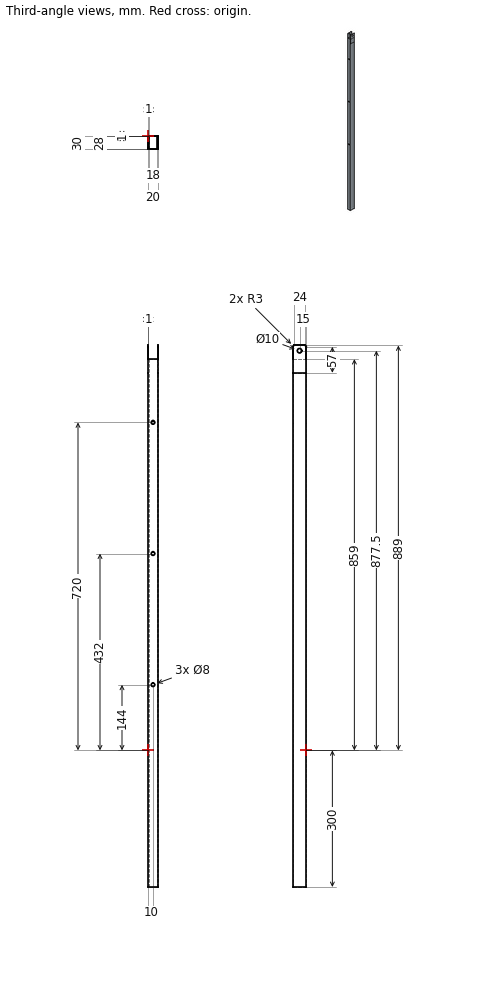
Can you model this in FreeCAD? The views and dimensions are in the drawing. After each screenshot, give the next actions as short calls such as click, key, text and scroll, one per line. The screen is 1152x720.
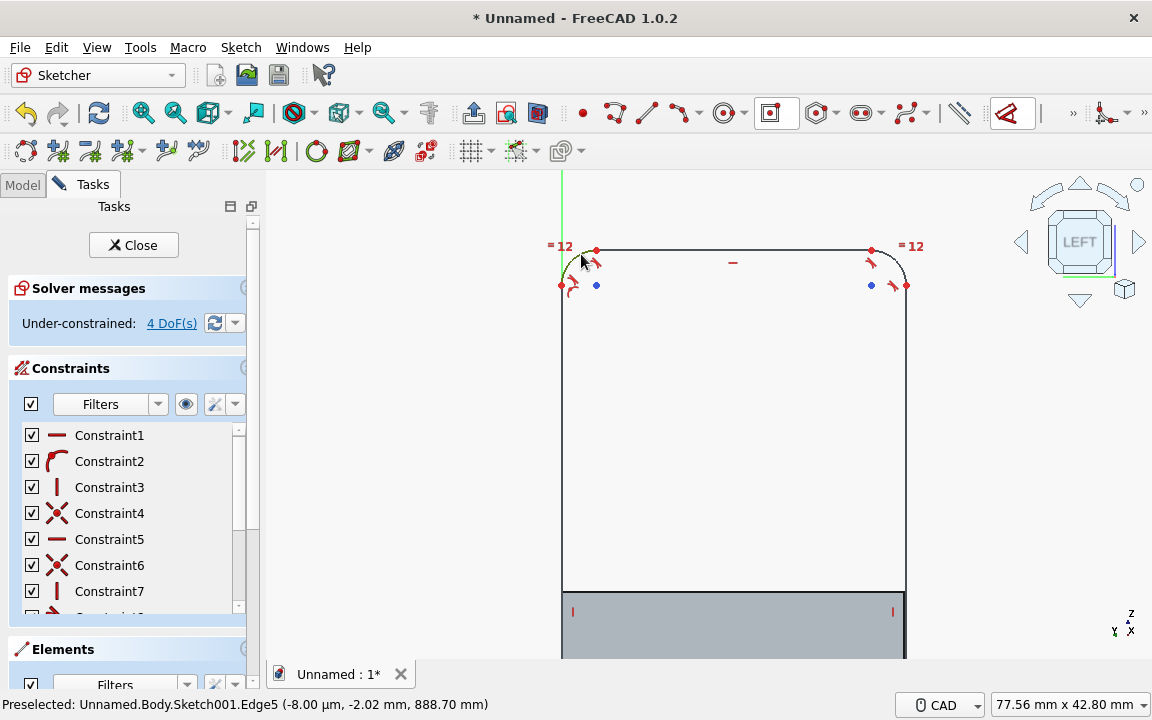
key(k)
key(r)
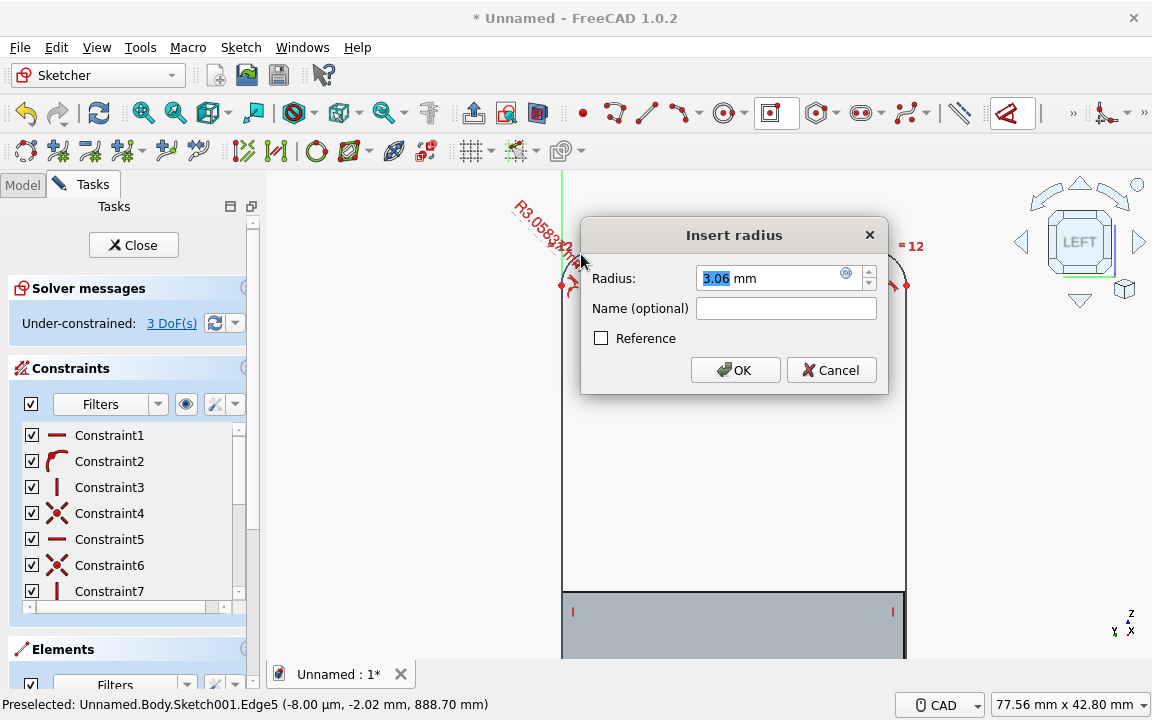
text(3)
key(Return)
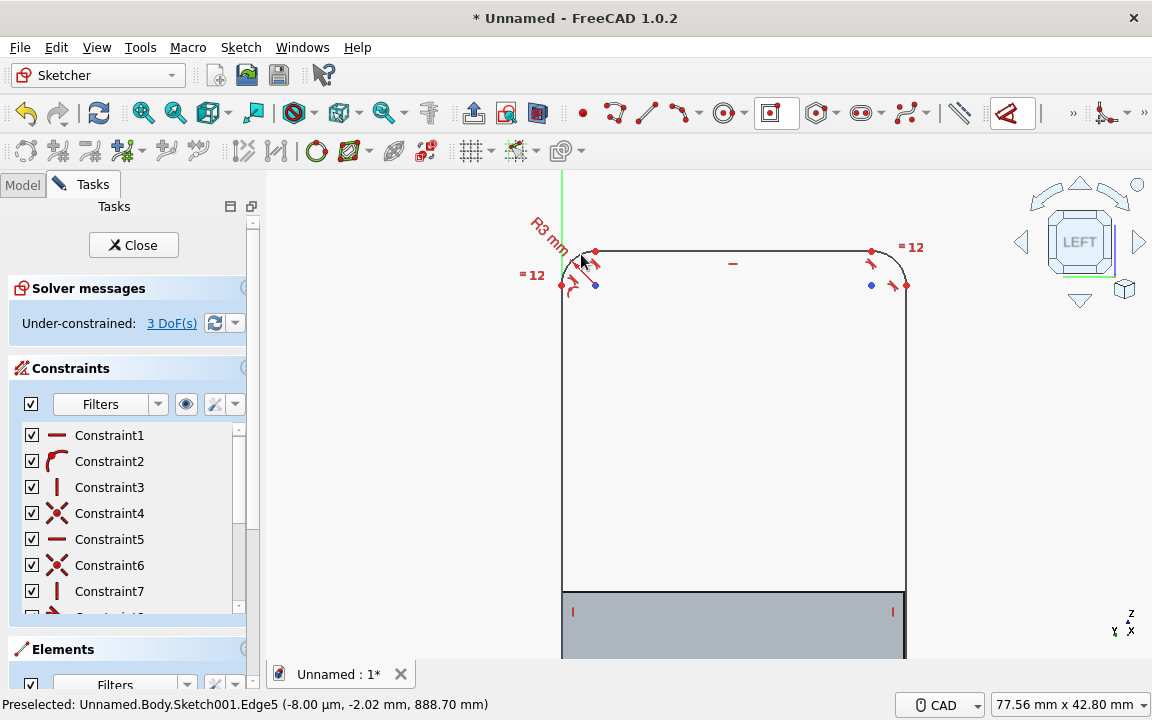
click(789, 251)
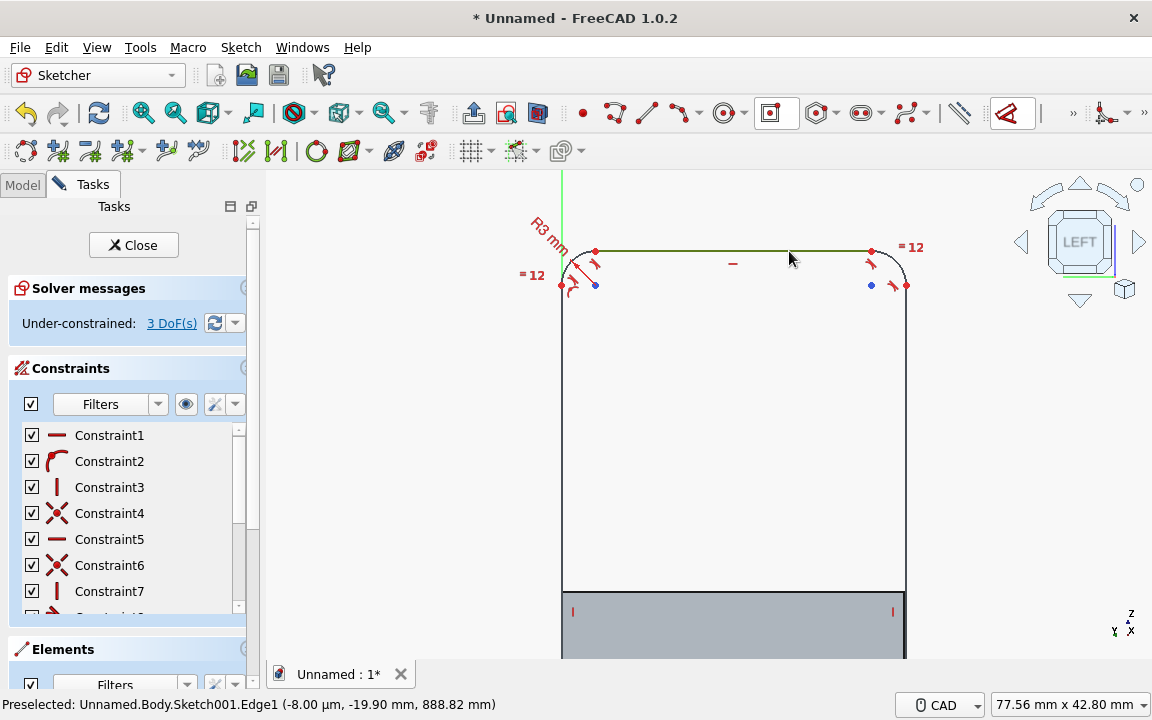
click(1030, 114)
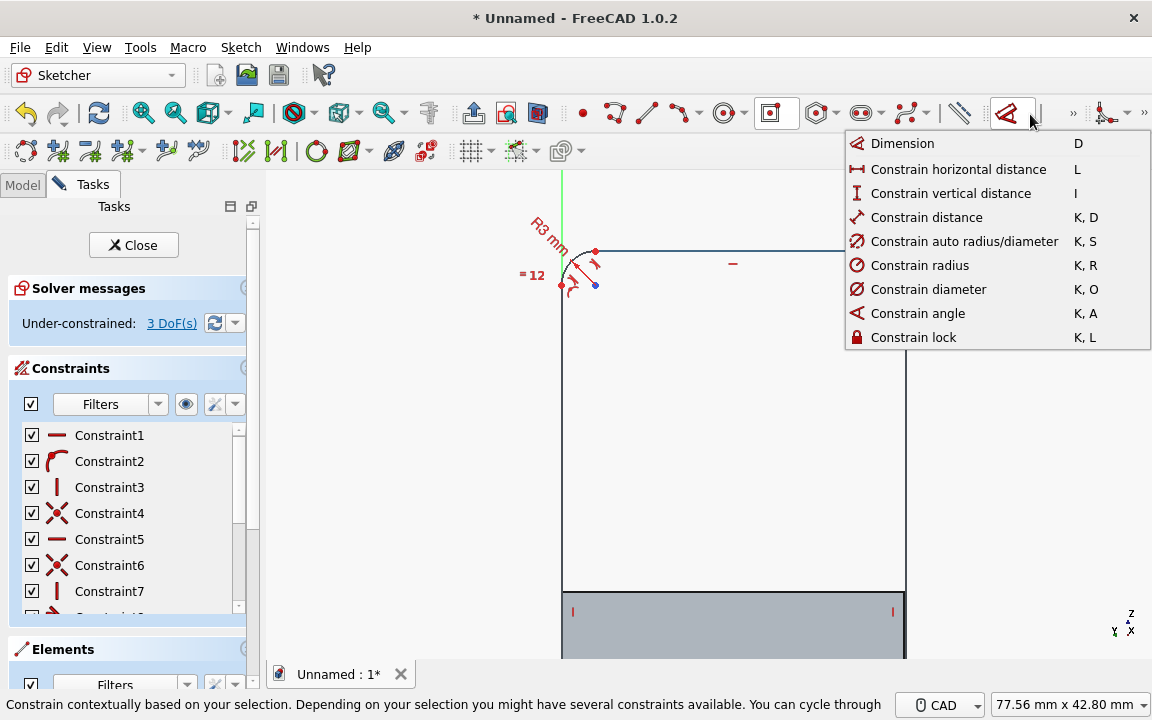
click(998, 169)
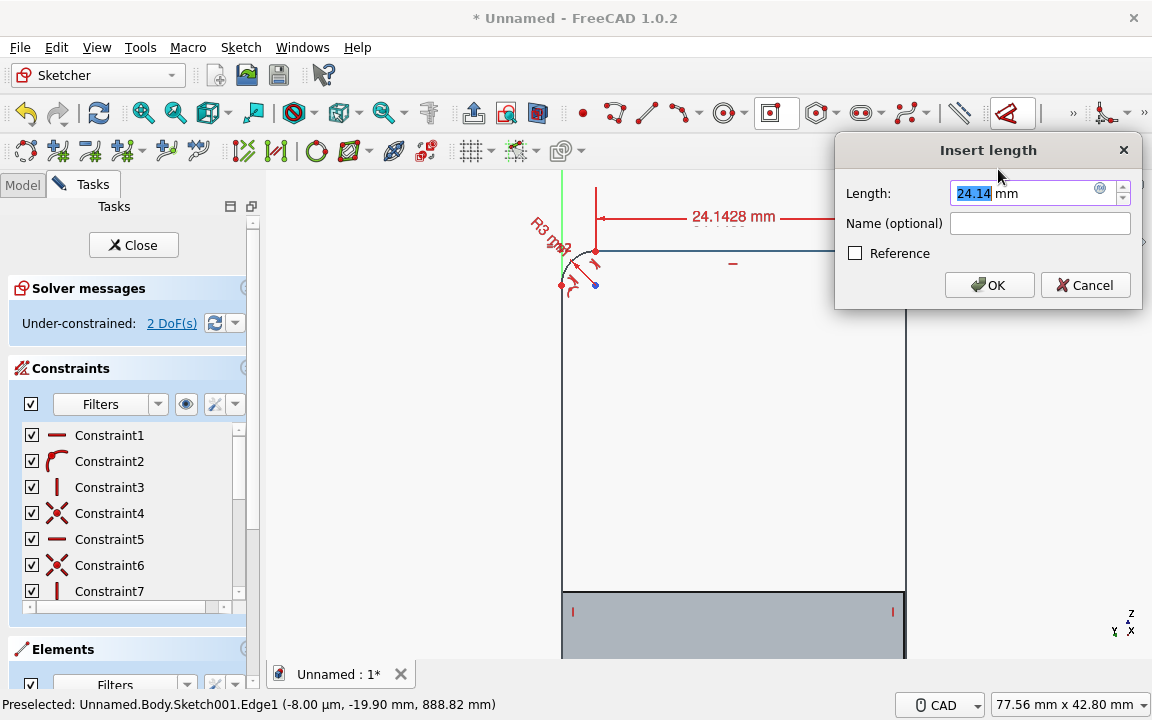
text(24)
key(Return)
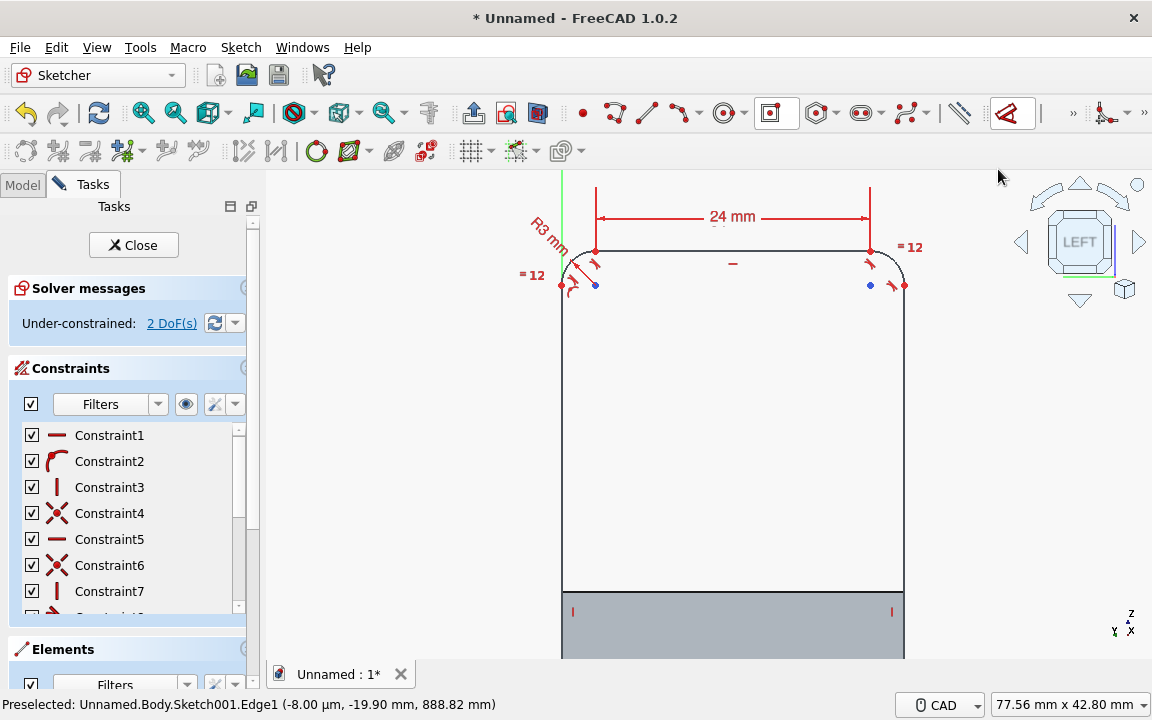
click(562, 481)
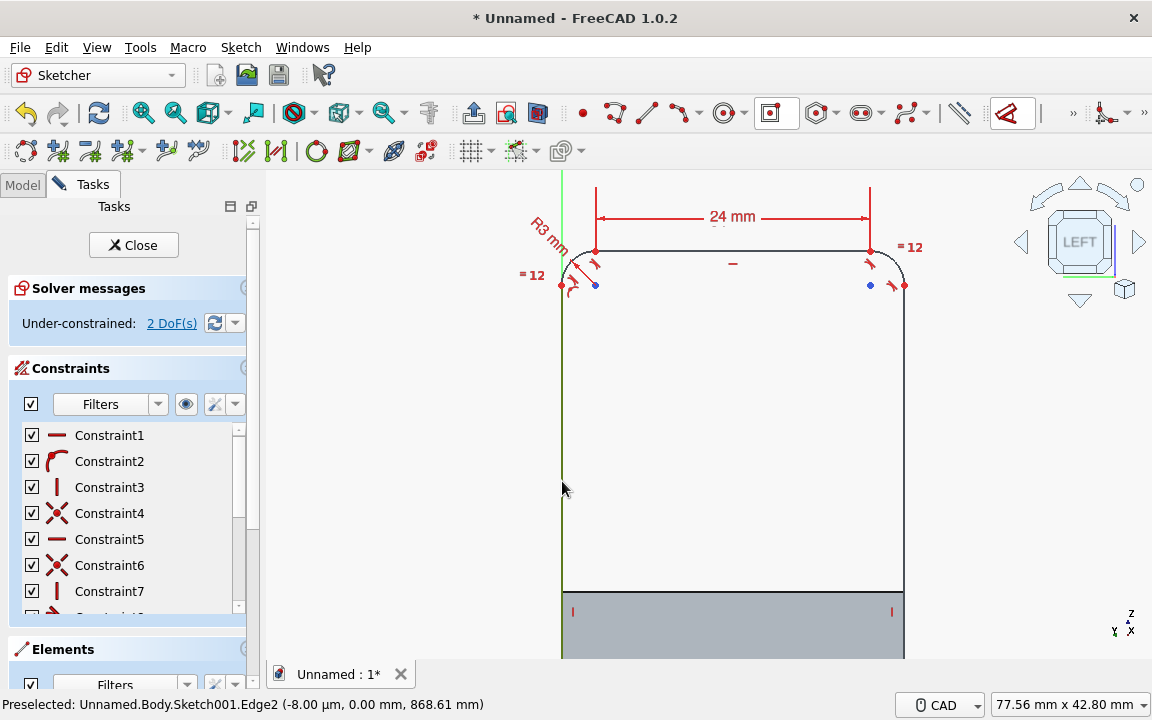
key(i)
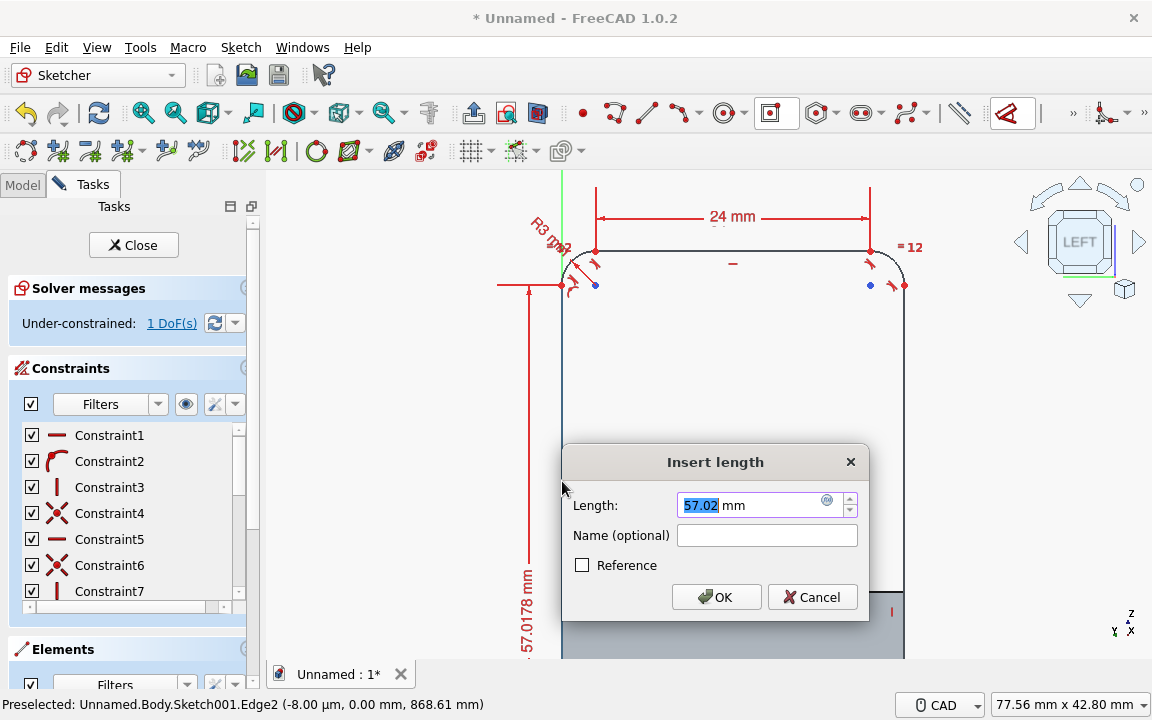
text(57)
key(Return)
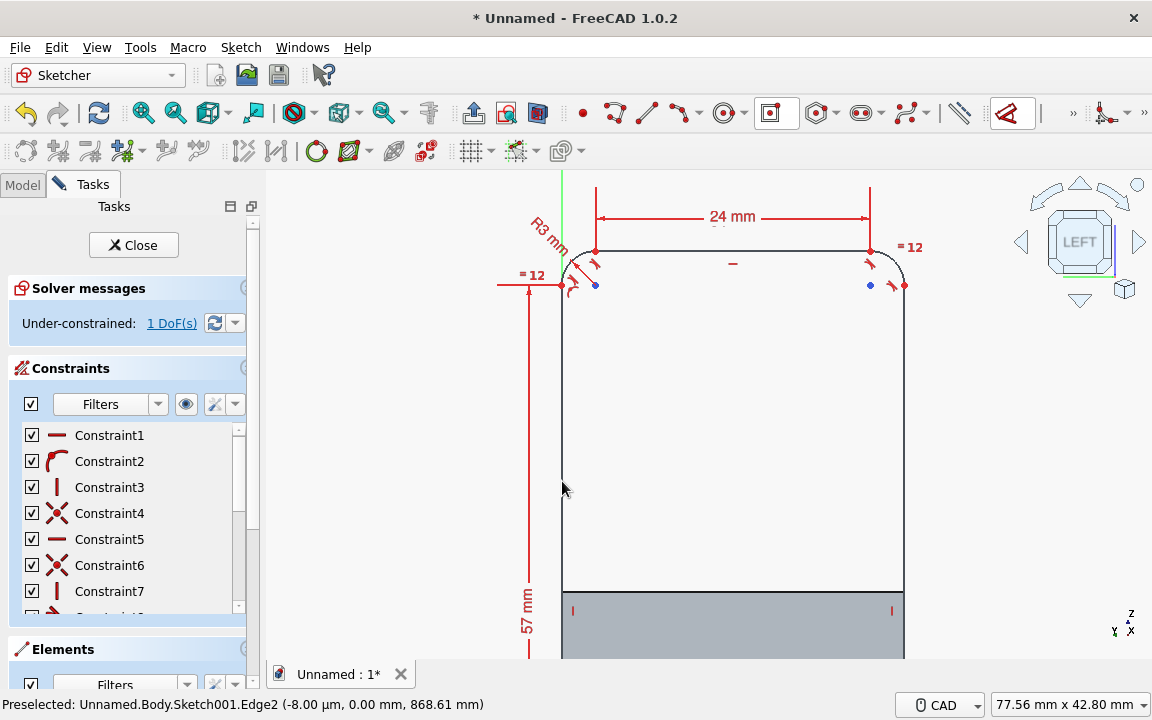
click(870, 251)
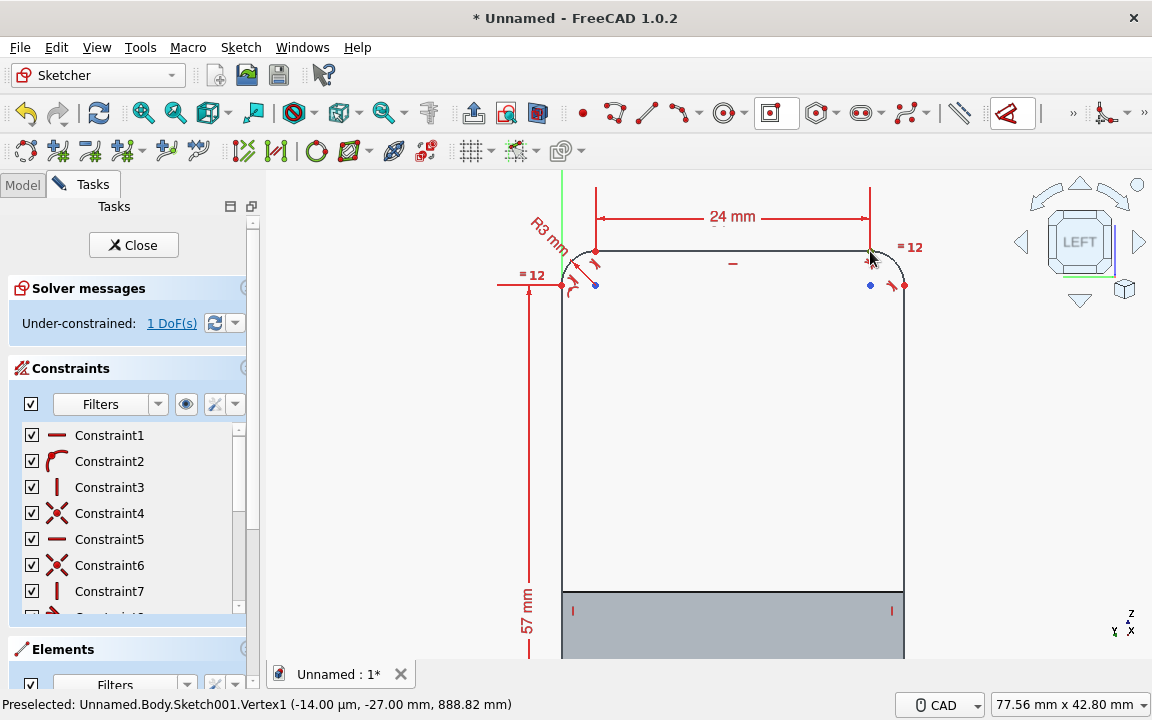
key(i)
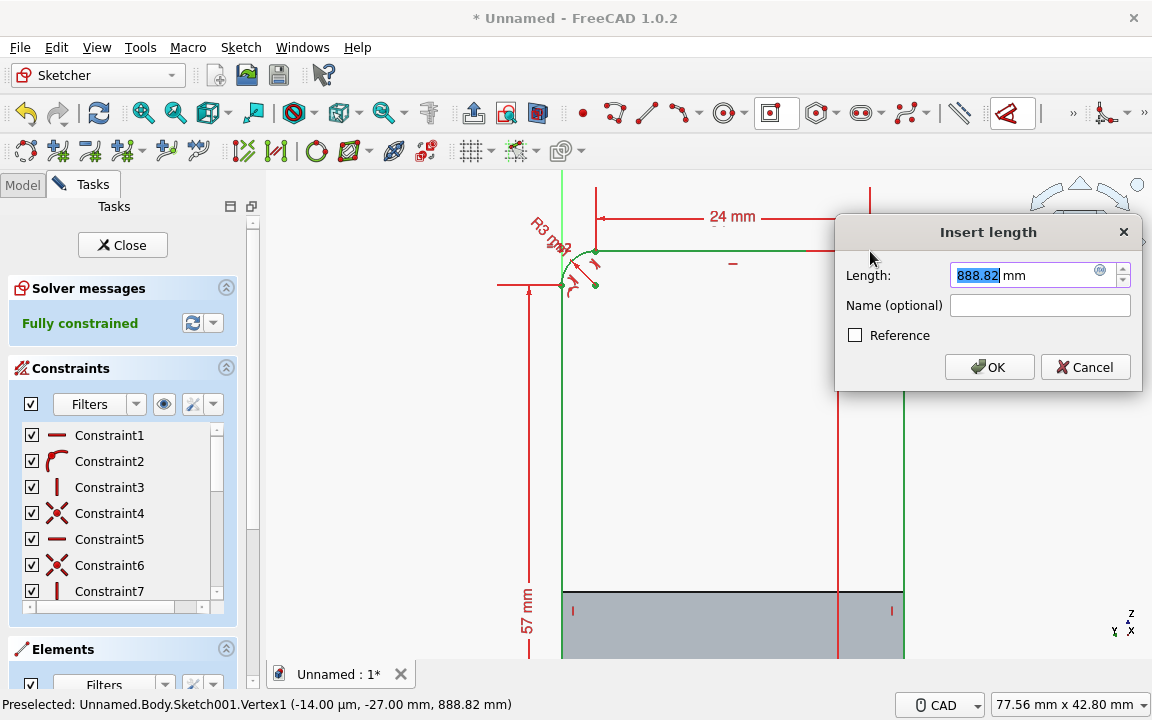
text(889)
key(Return)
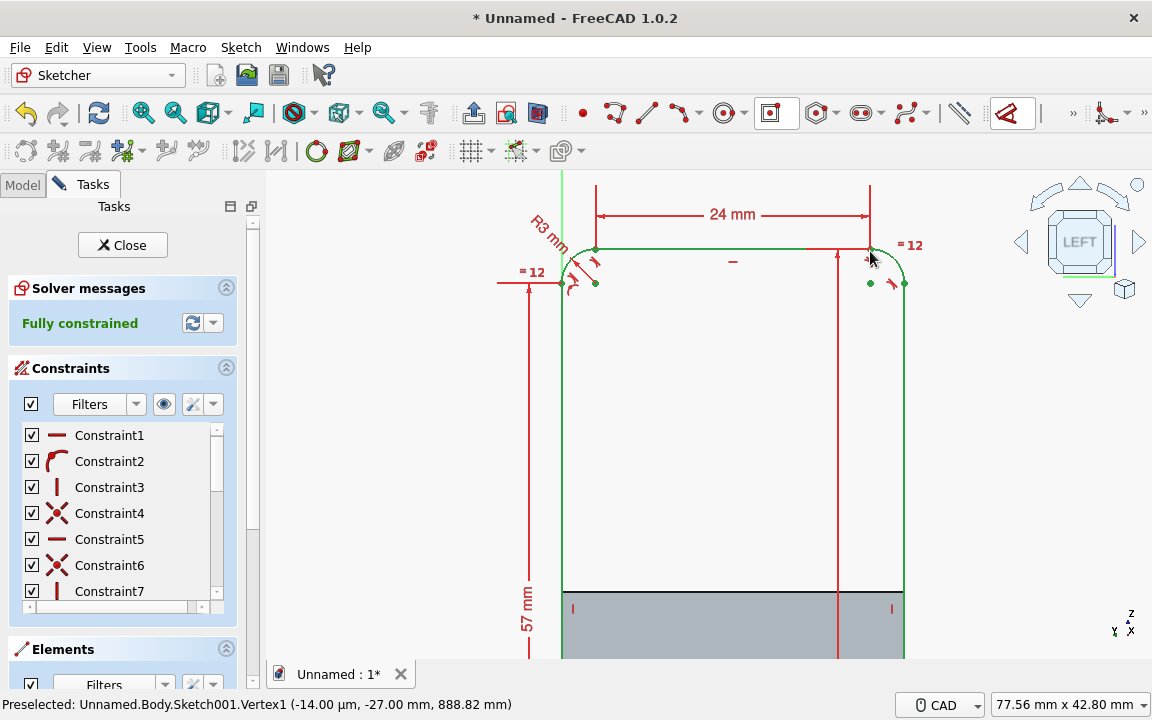
click(123, 245)